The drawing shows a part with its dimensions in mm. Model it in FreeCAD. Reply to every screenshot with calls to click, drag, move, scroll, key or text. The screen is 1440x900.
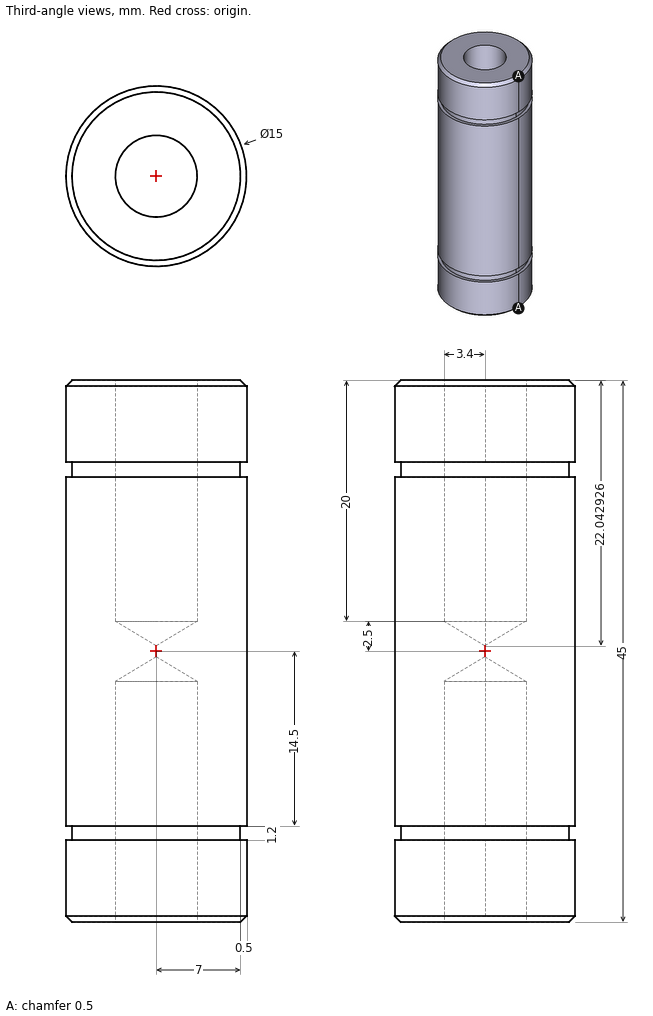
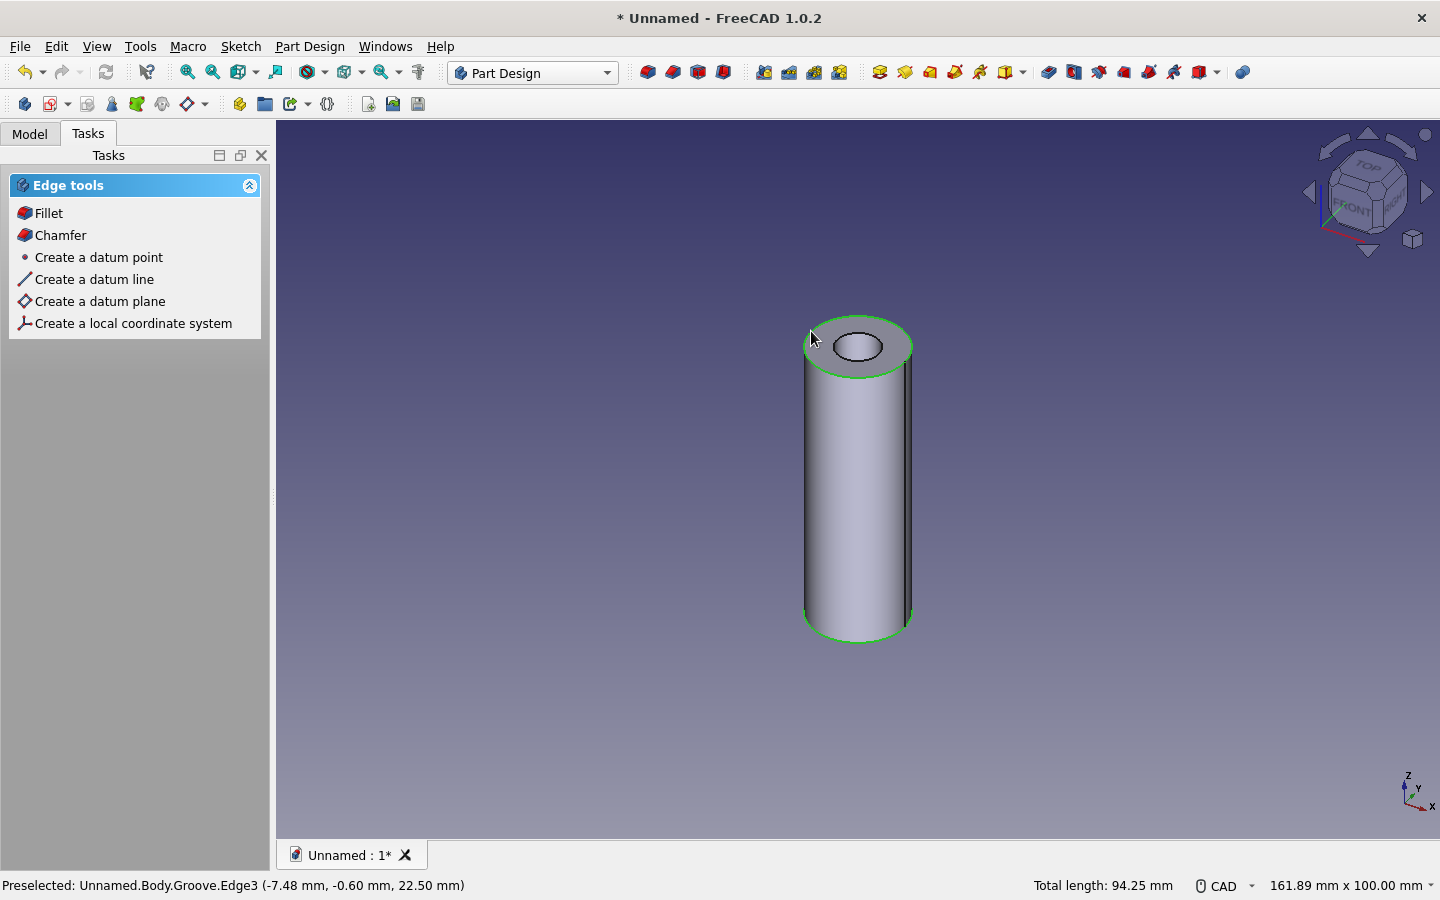
click(673, 72)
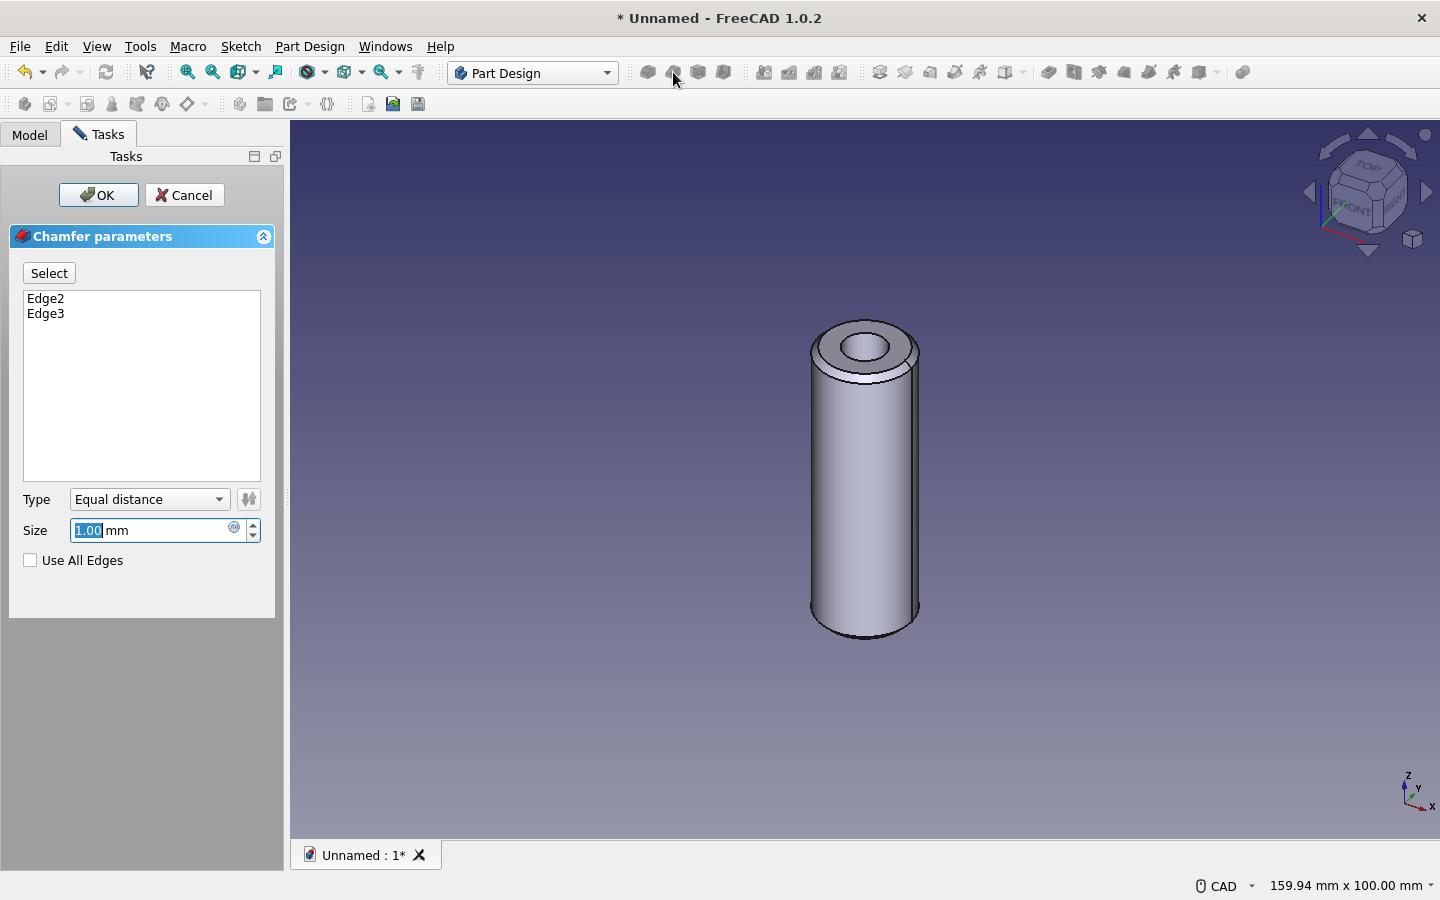
text(0.5)
key(Tab)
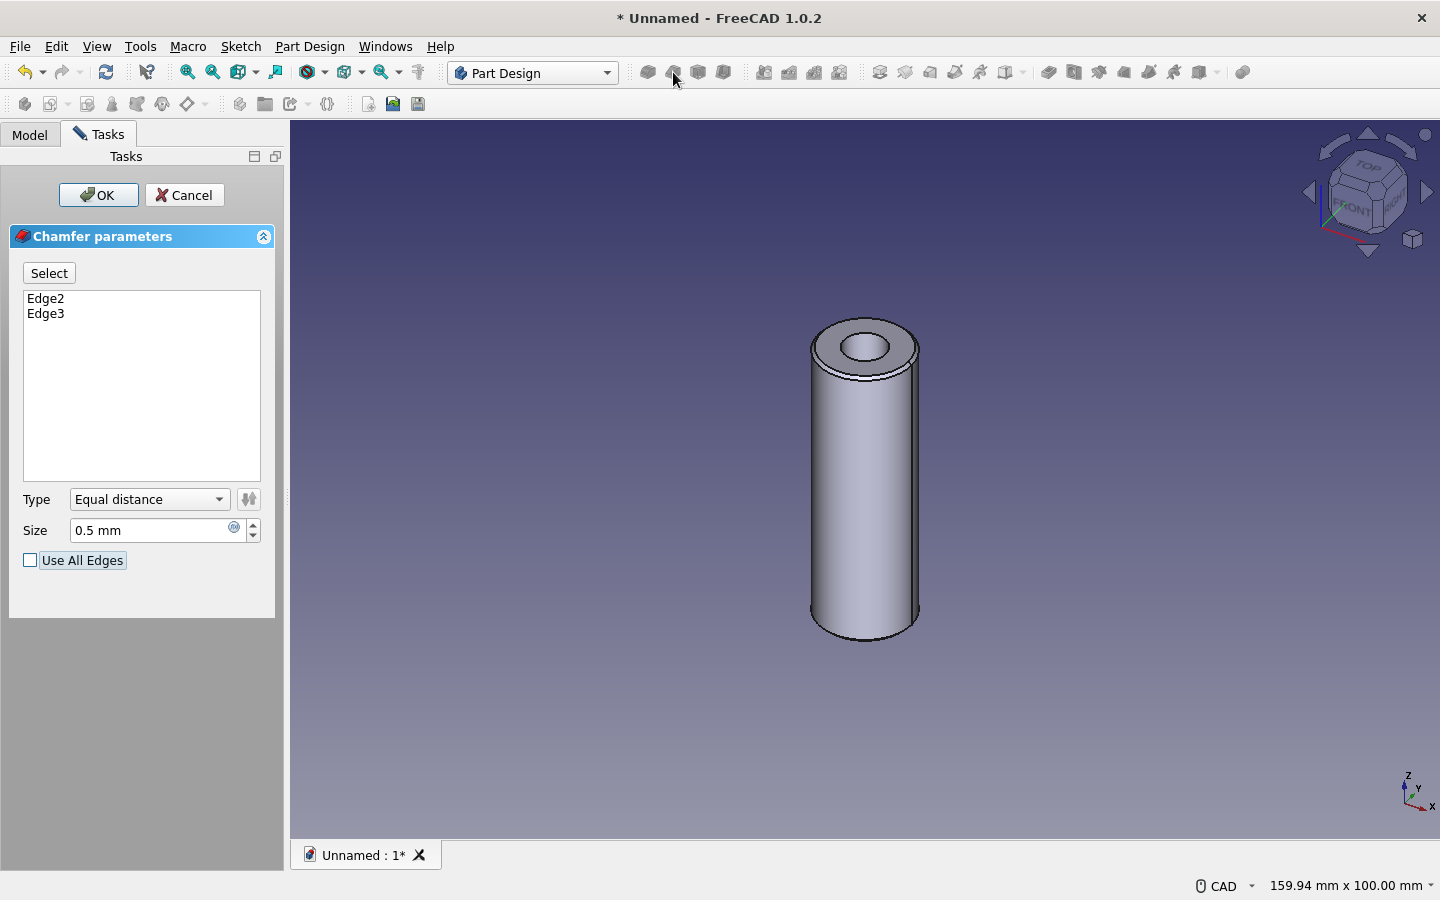
click(99, 195)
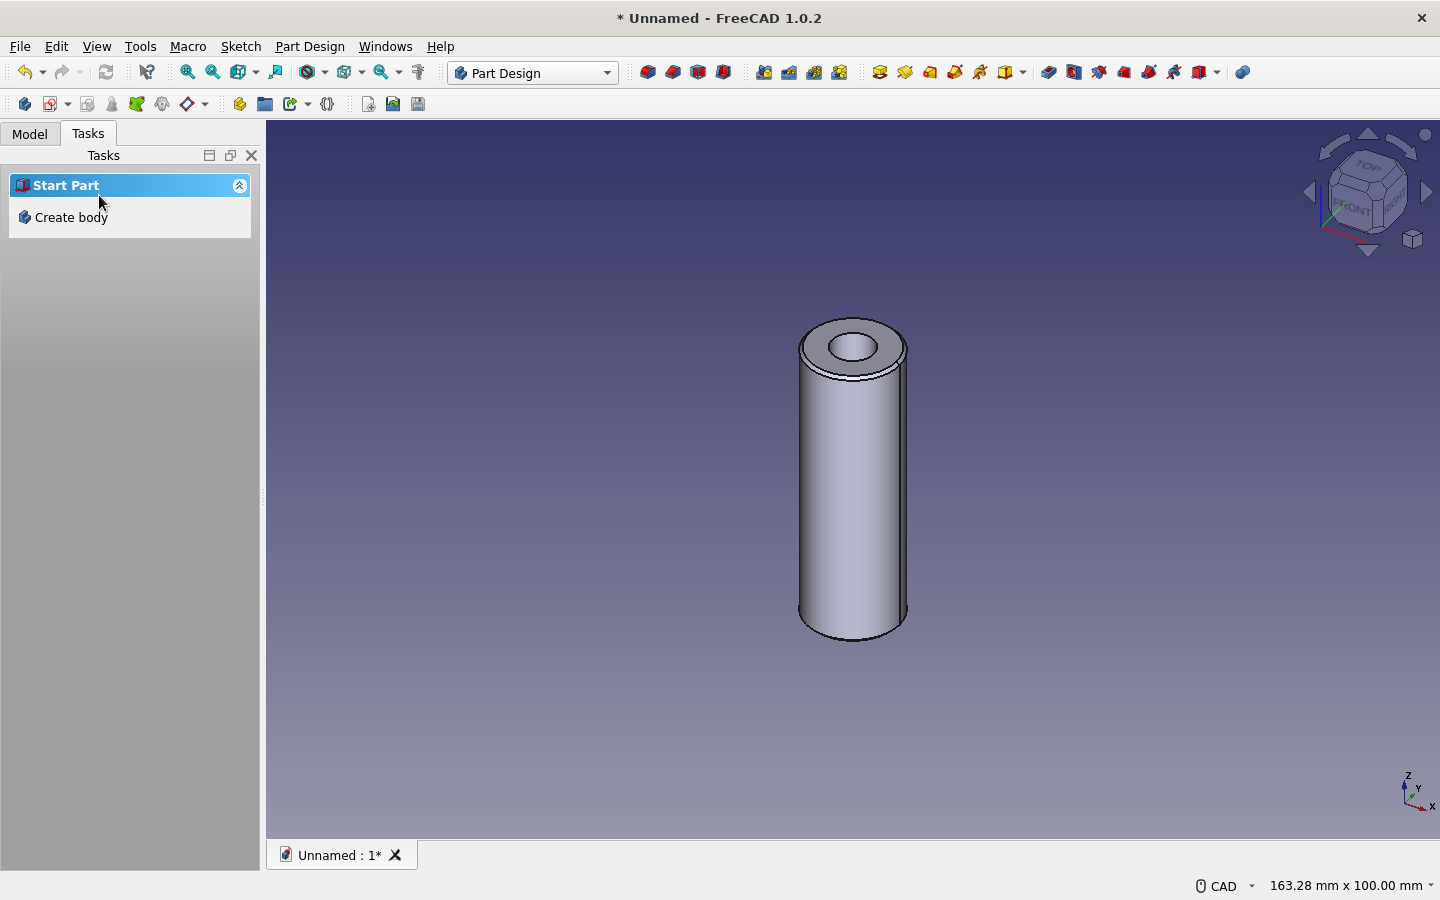
click(30, 134)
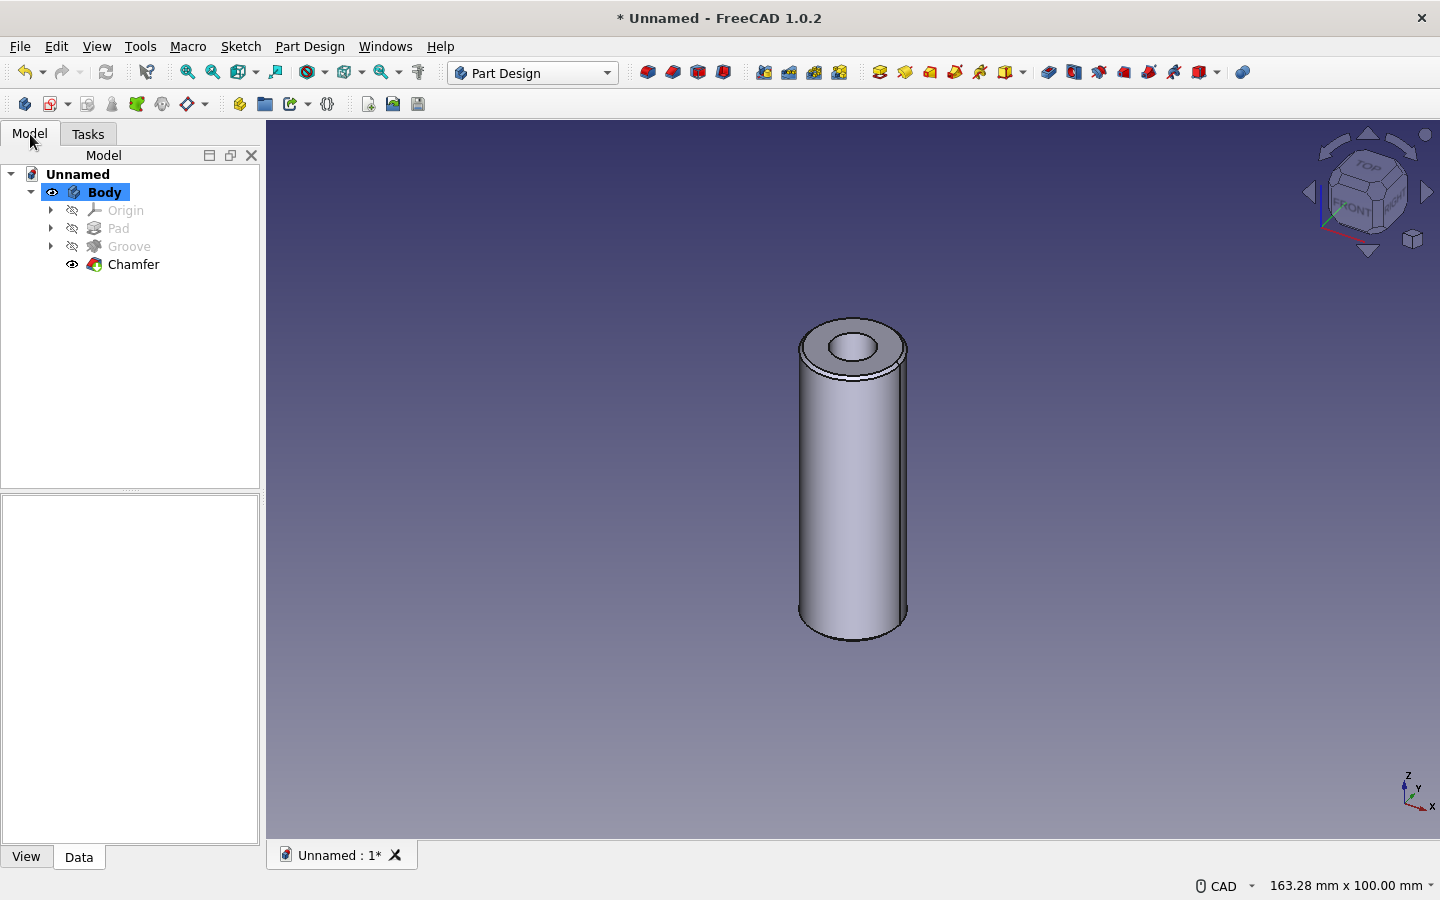
click(117, 246)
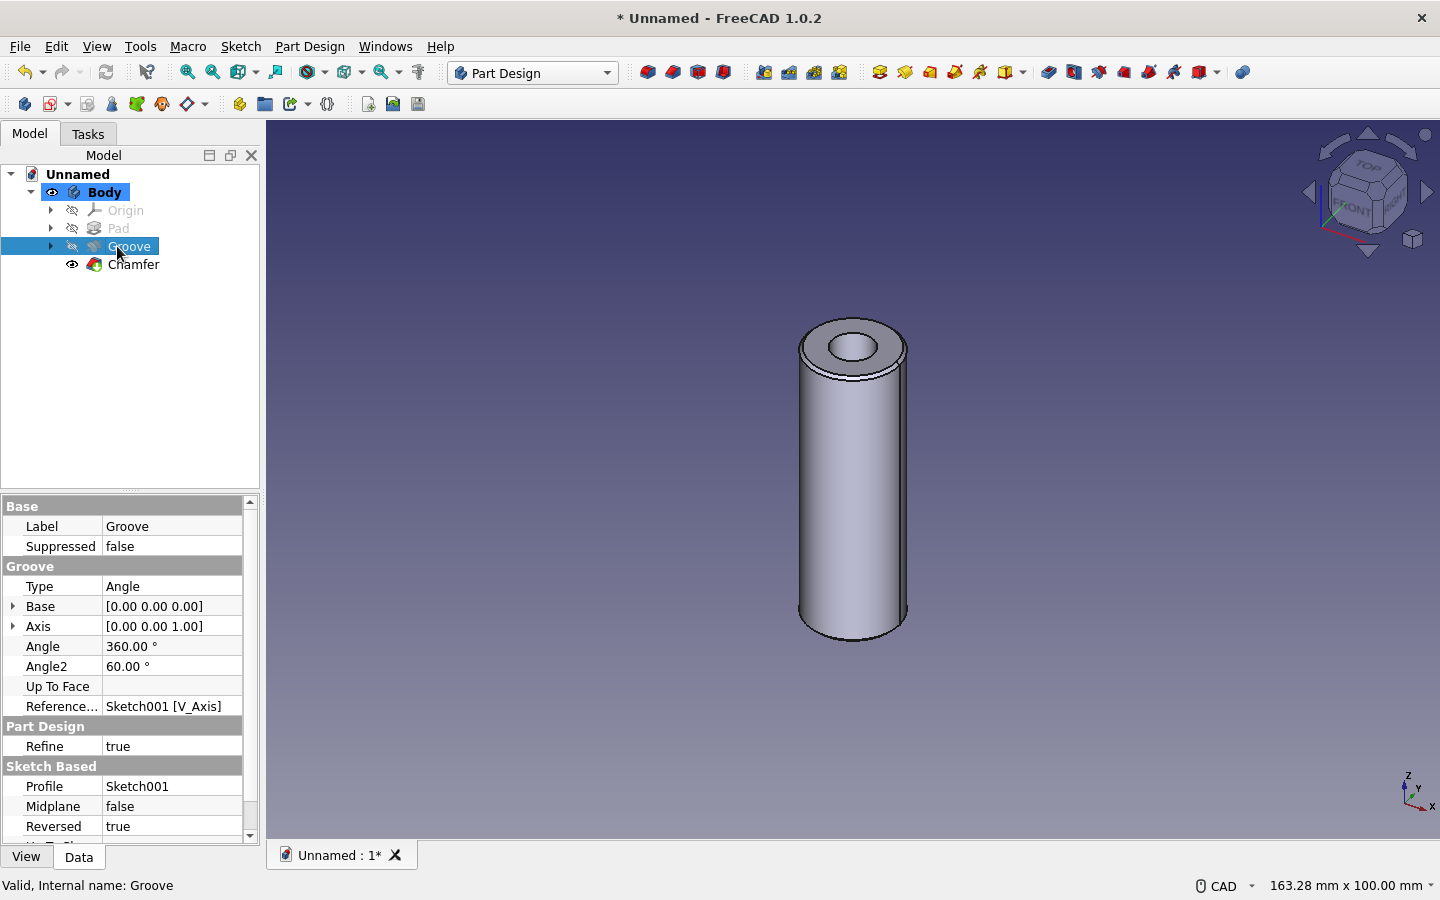
click(764, 72)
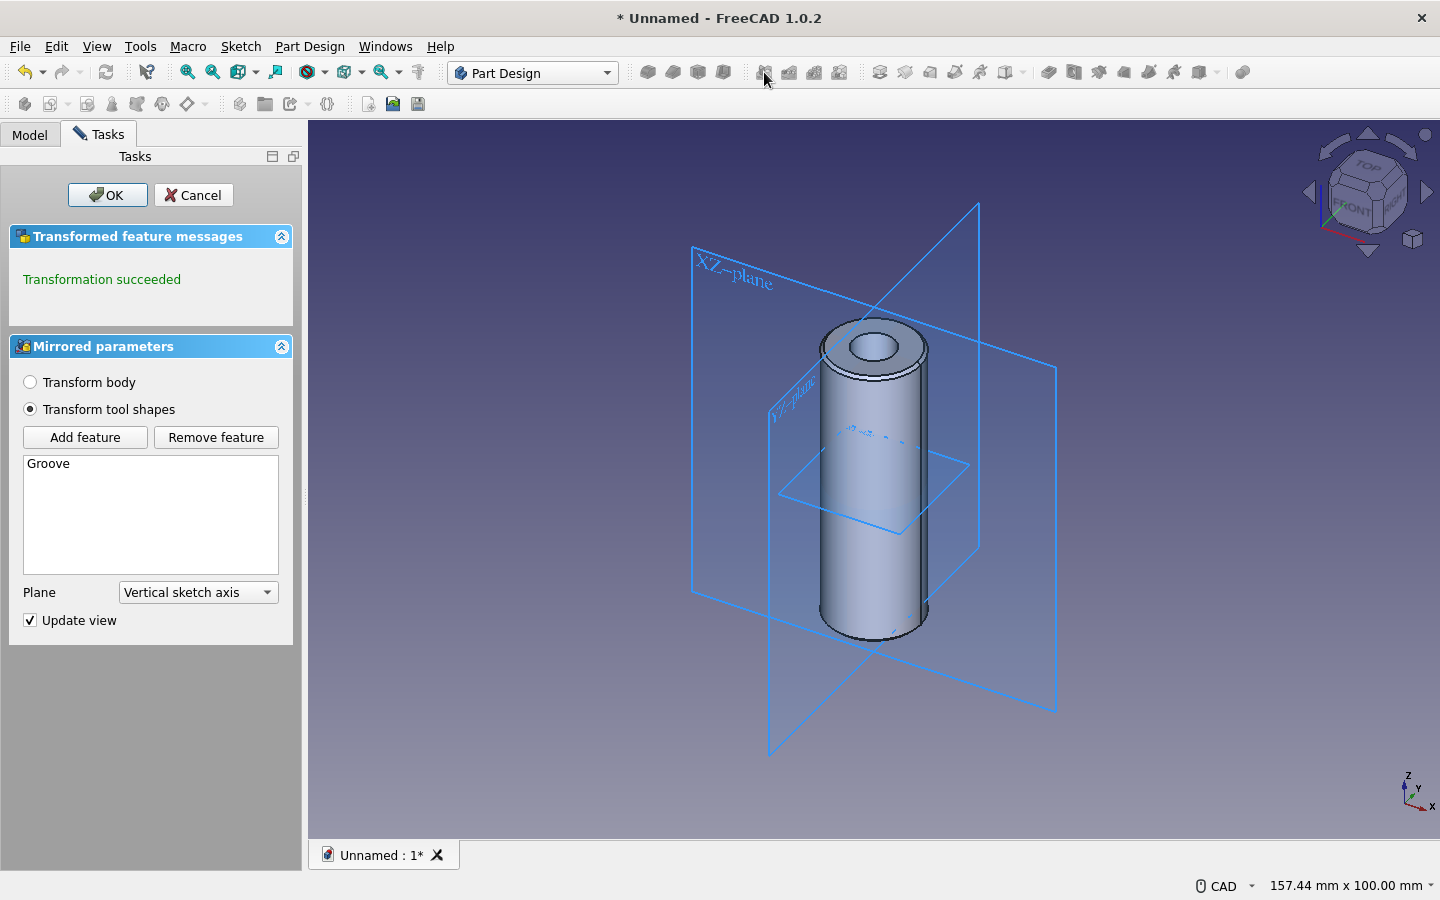
click(199, 592)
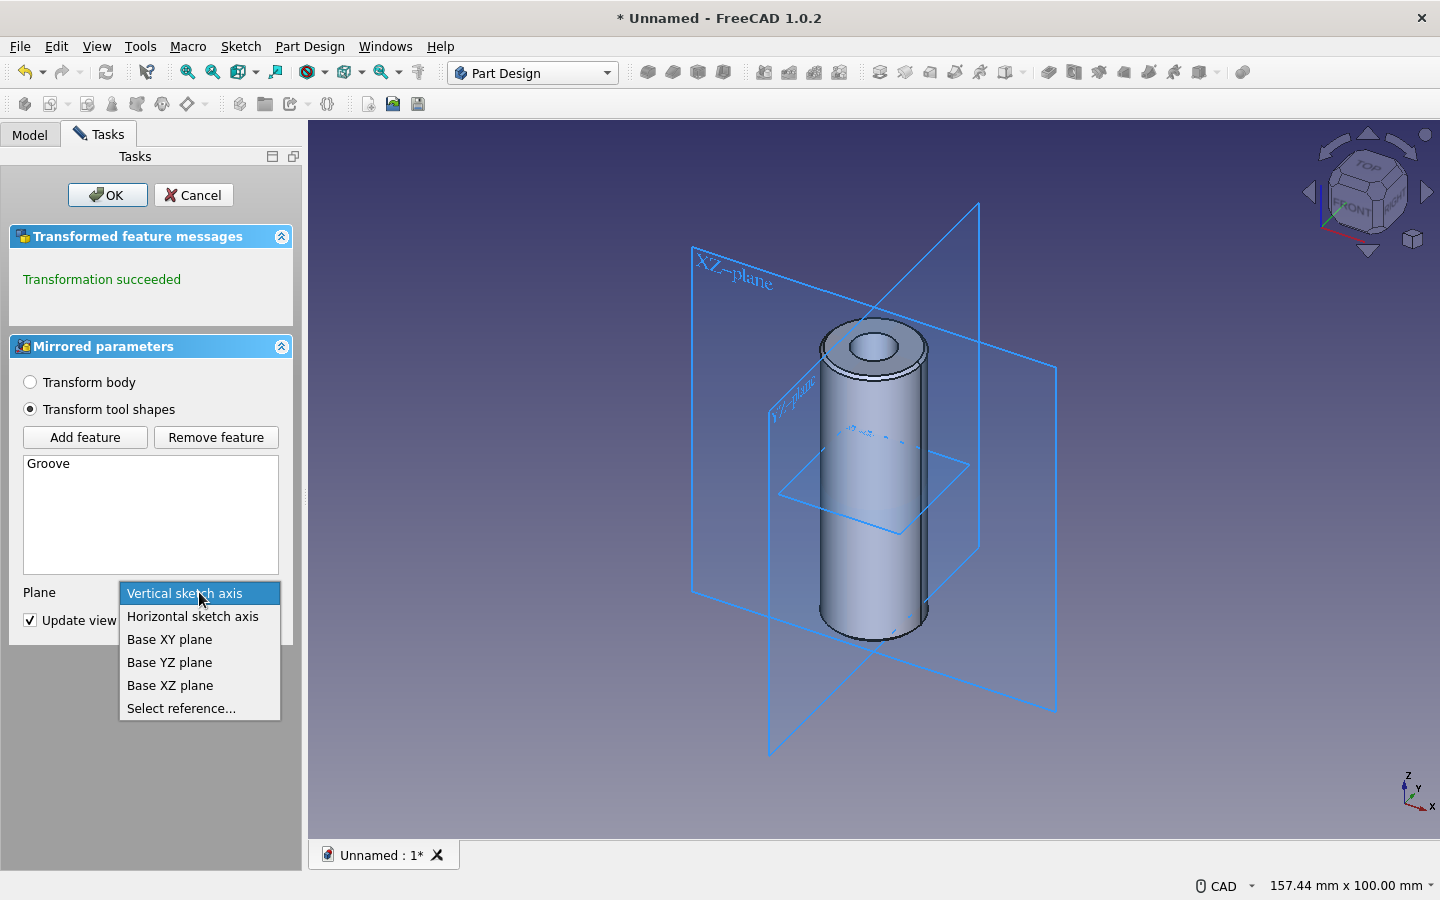
click(198, 640)